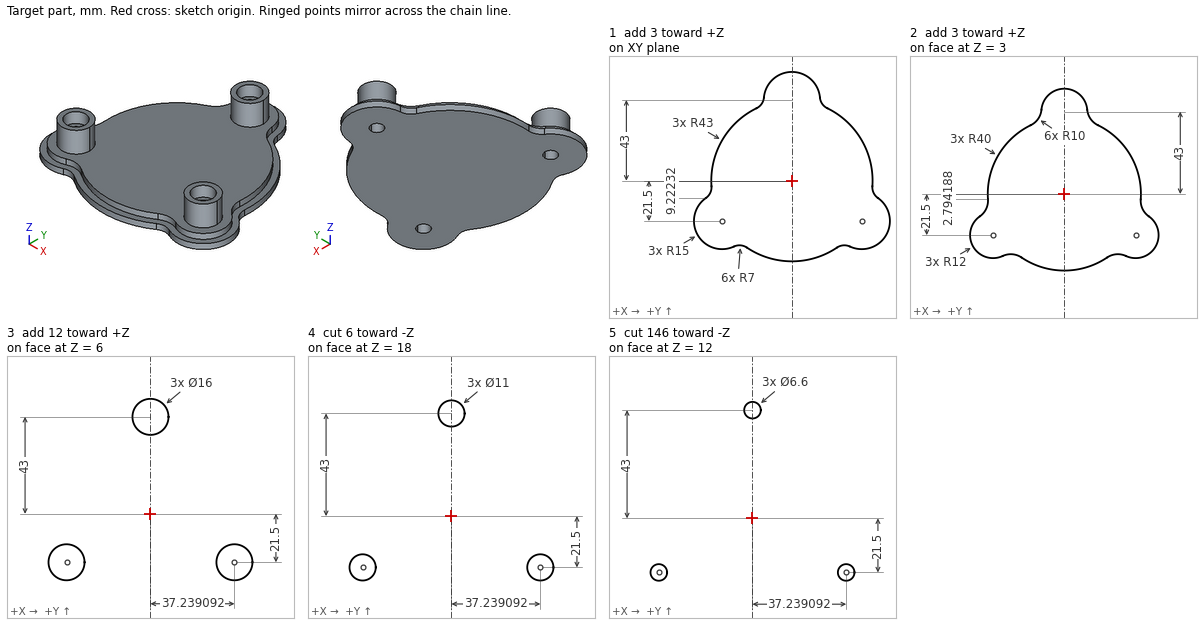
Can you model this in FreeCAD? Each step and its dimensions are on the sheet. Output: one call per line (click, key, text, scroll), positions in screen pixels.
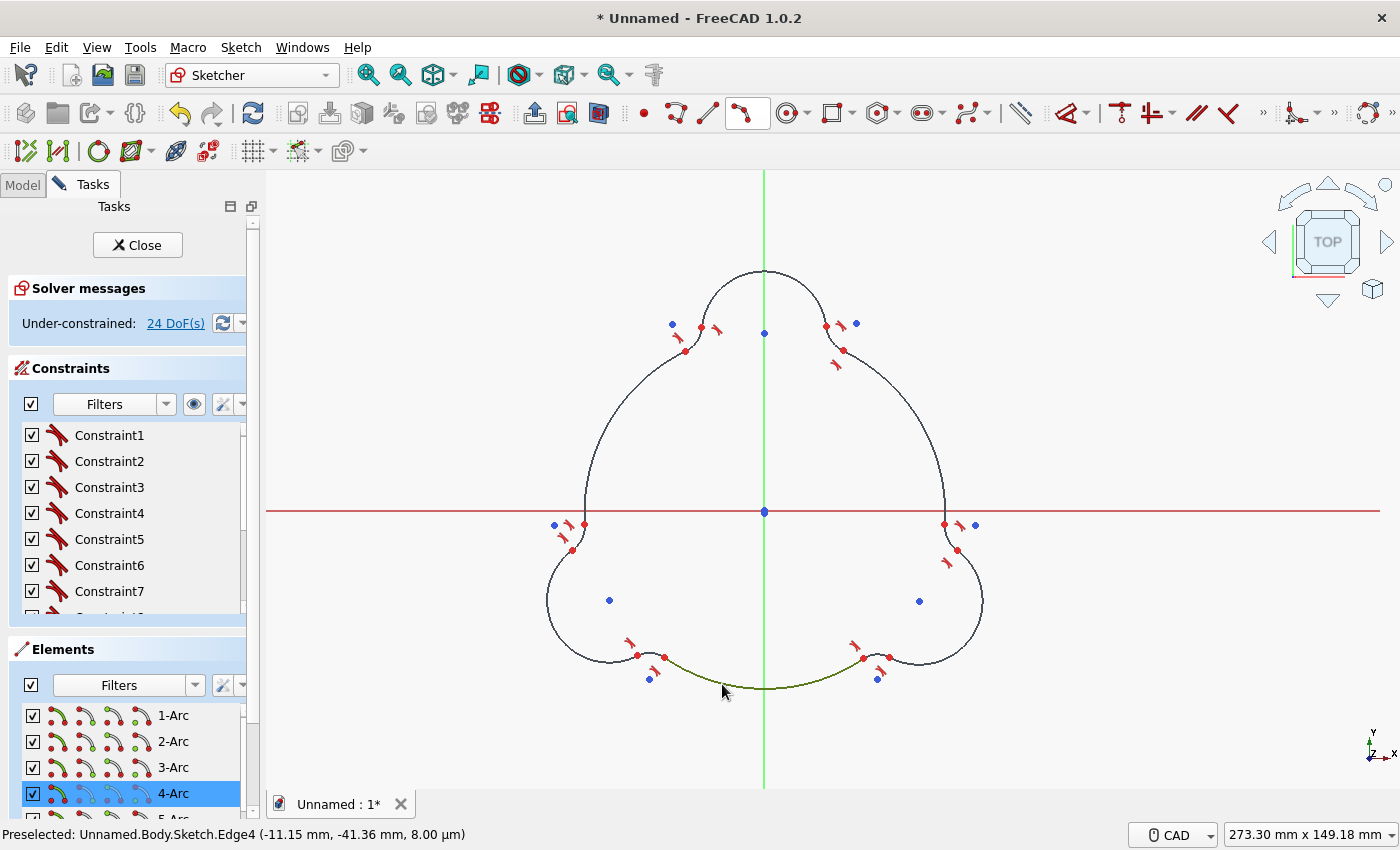
click(937, 461)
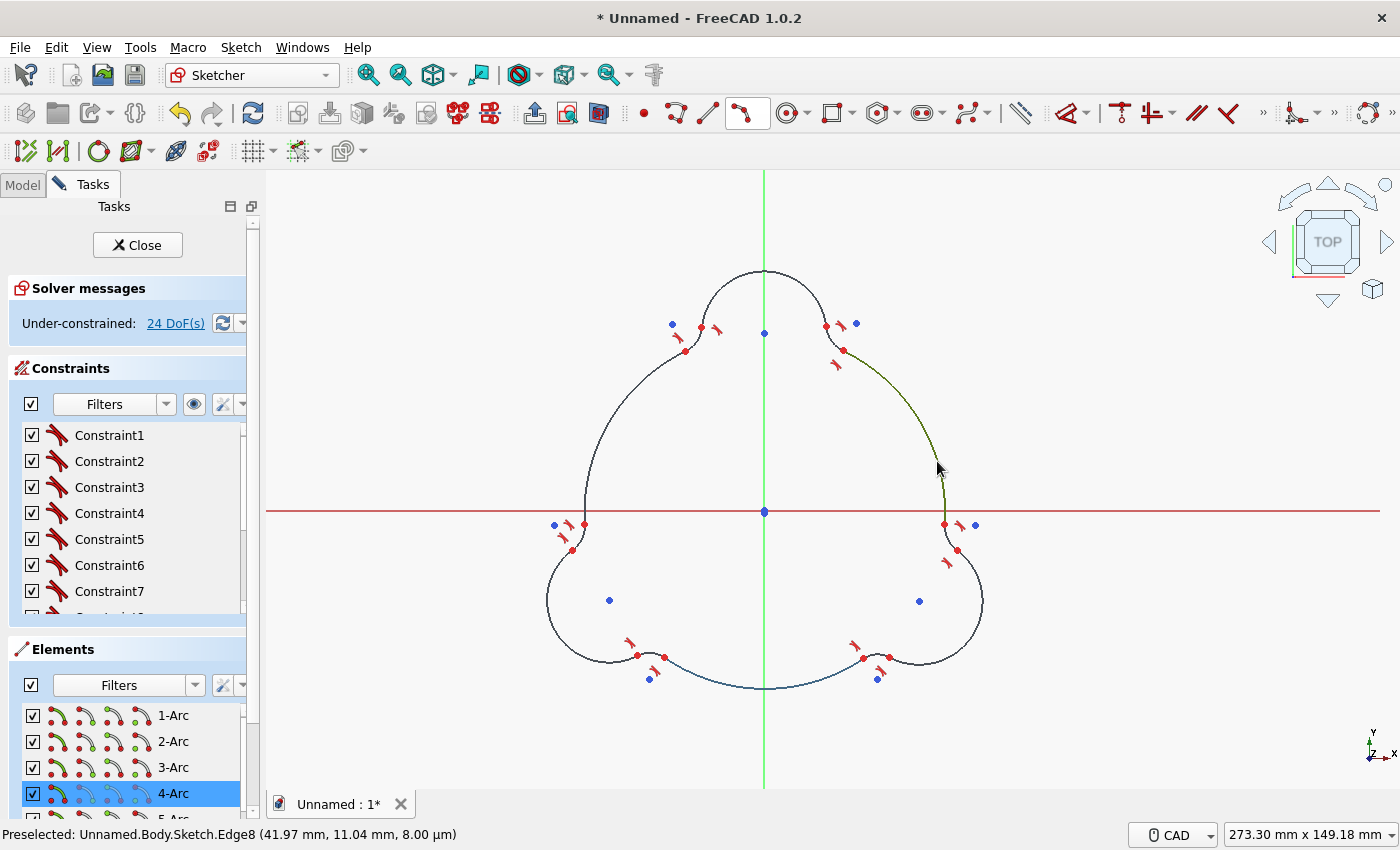
click(1120, 114)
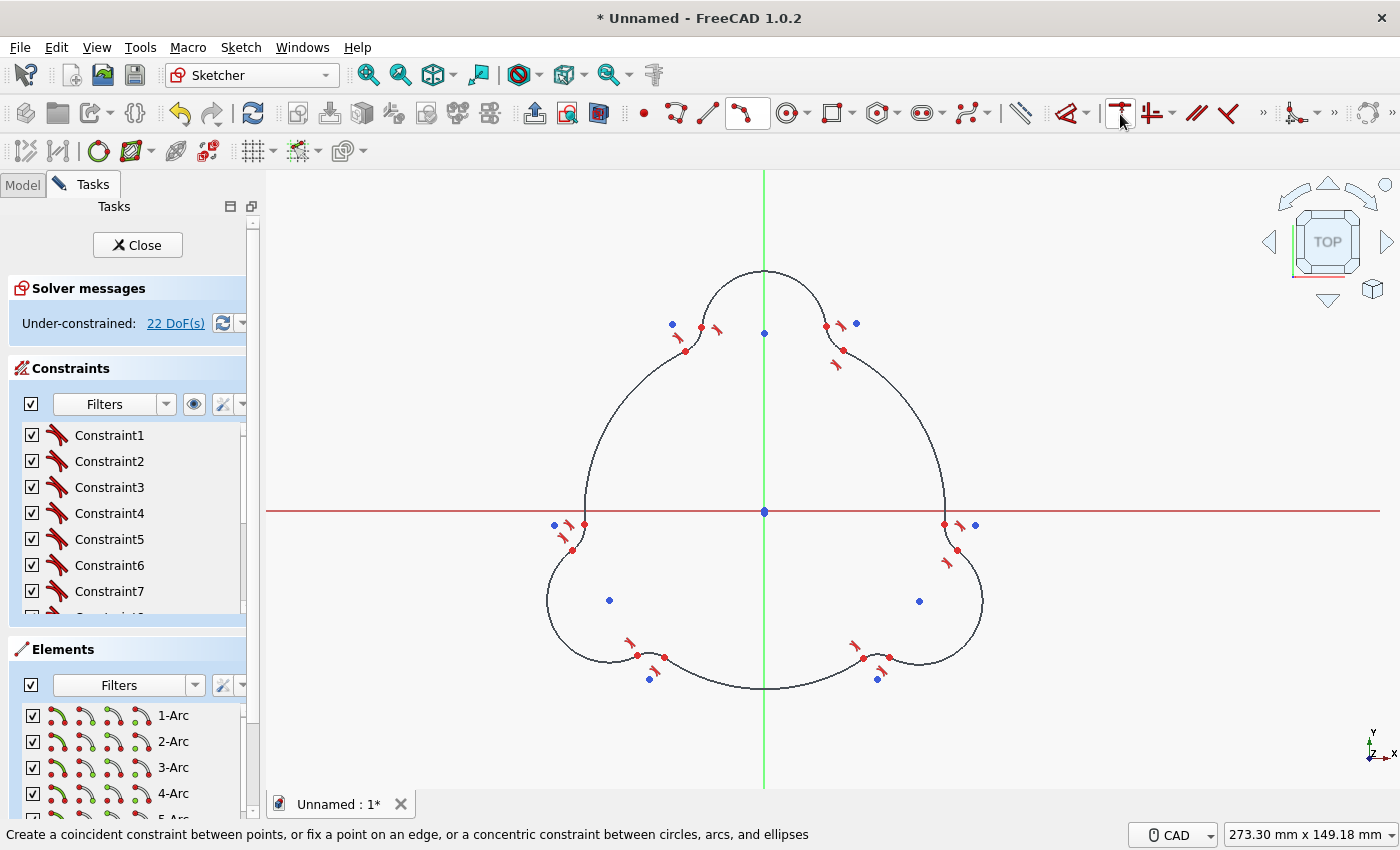
click(722, 684)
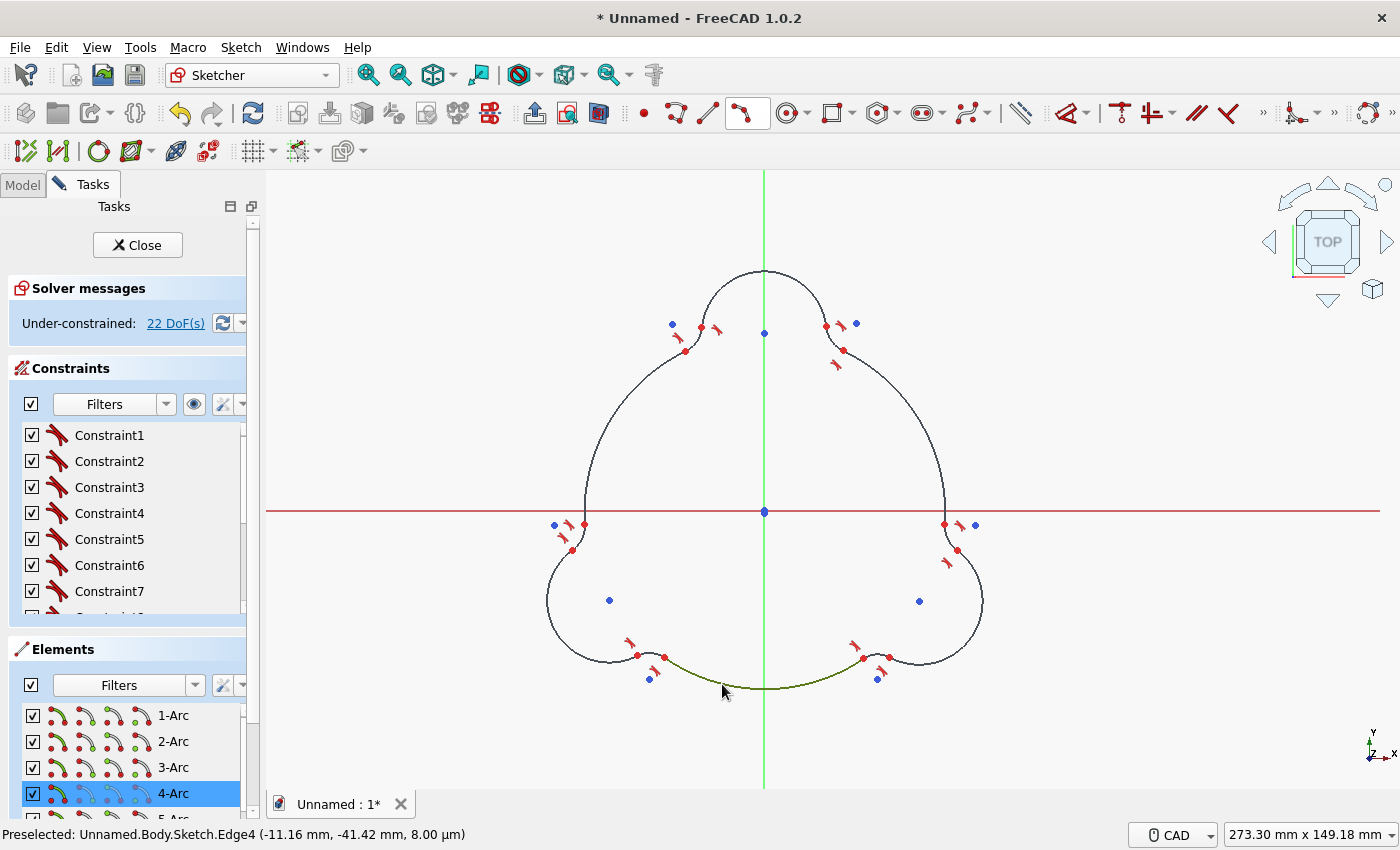
click(634, 389)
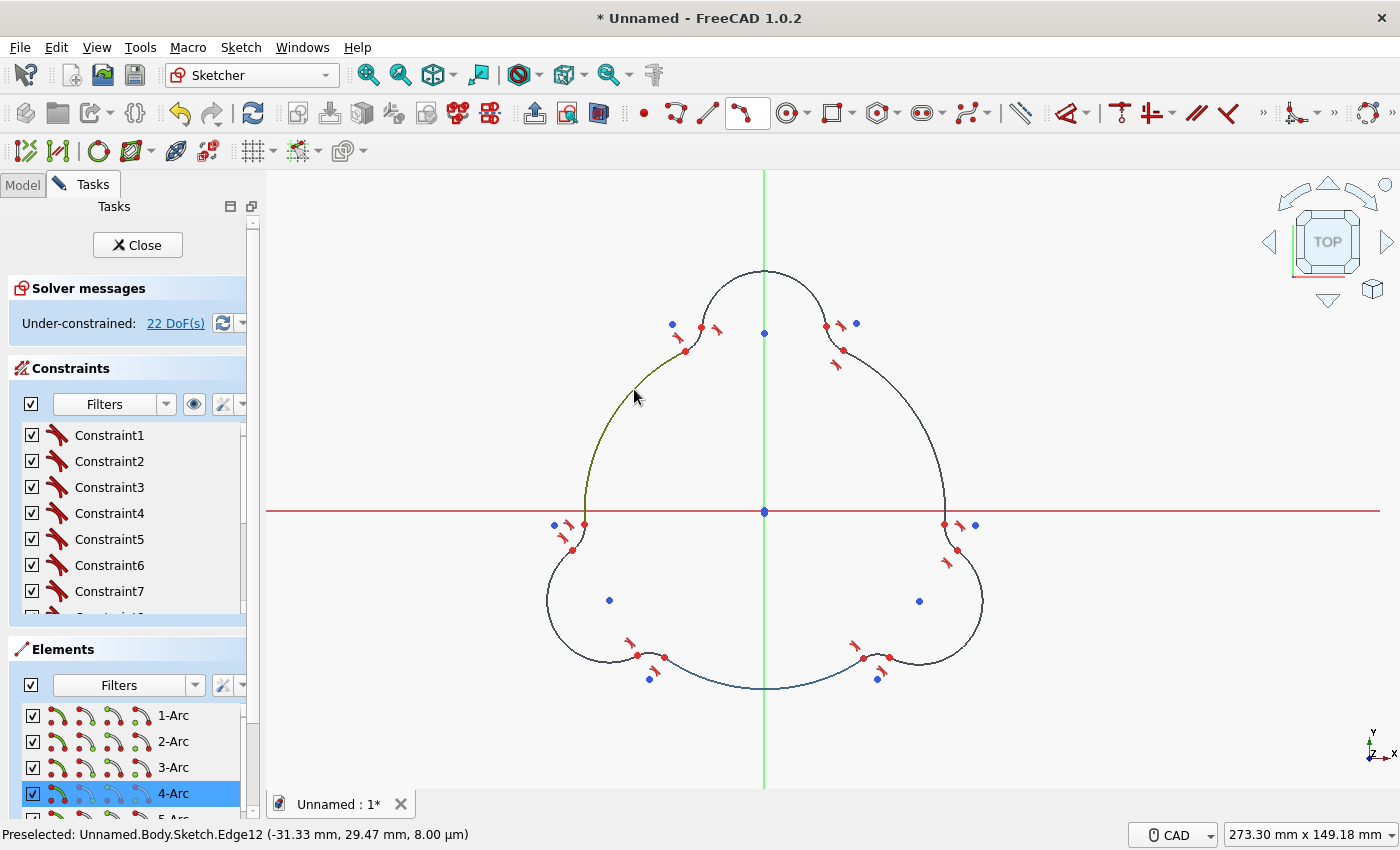
click(1120, 114)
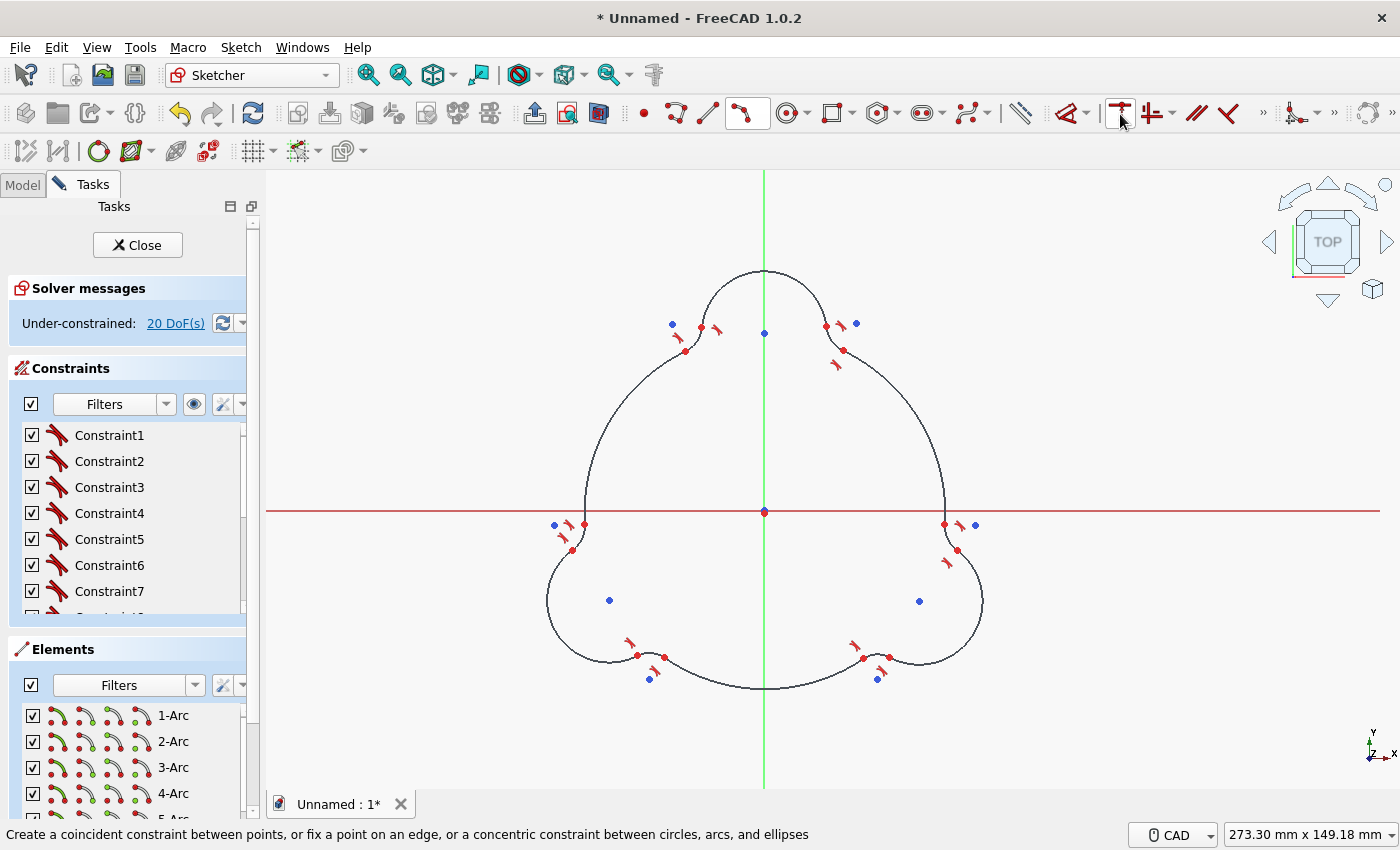
scroll(765, 512, up, 3)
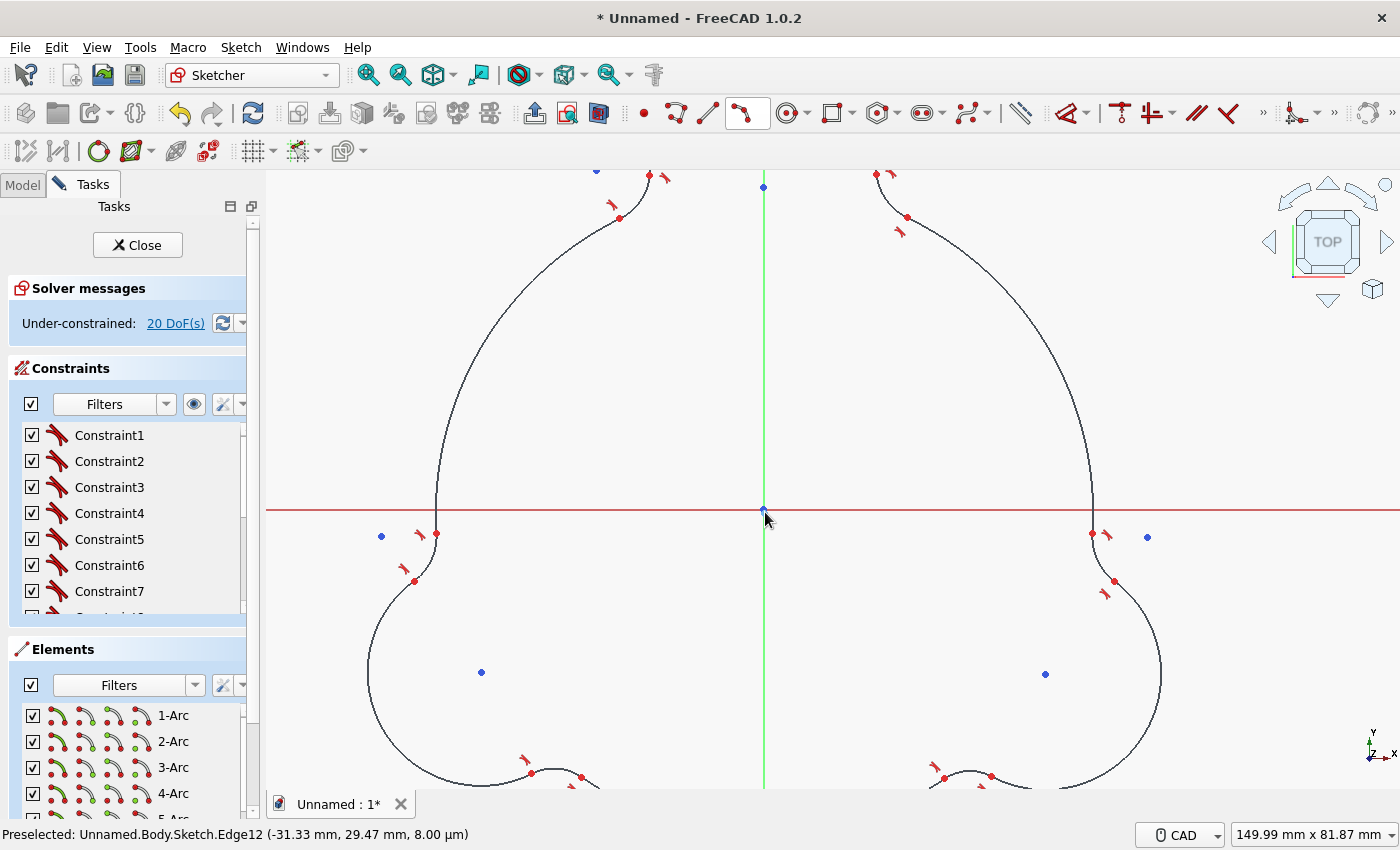
drag(754, 500, 774, 524)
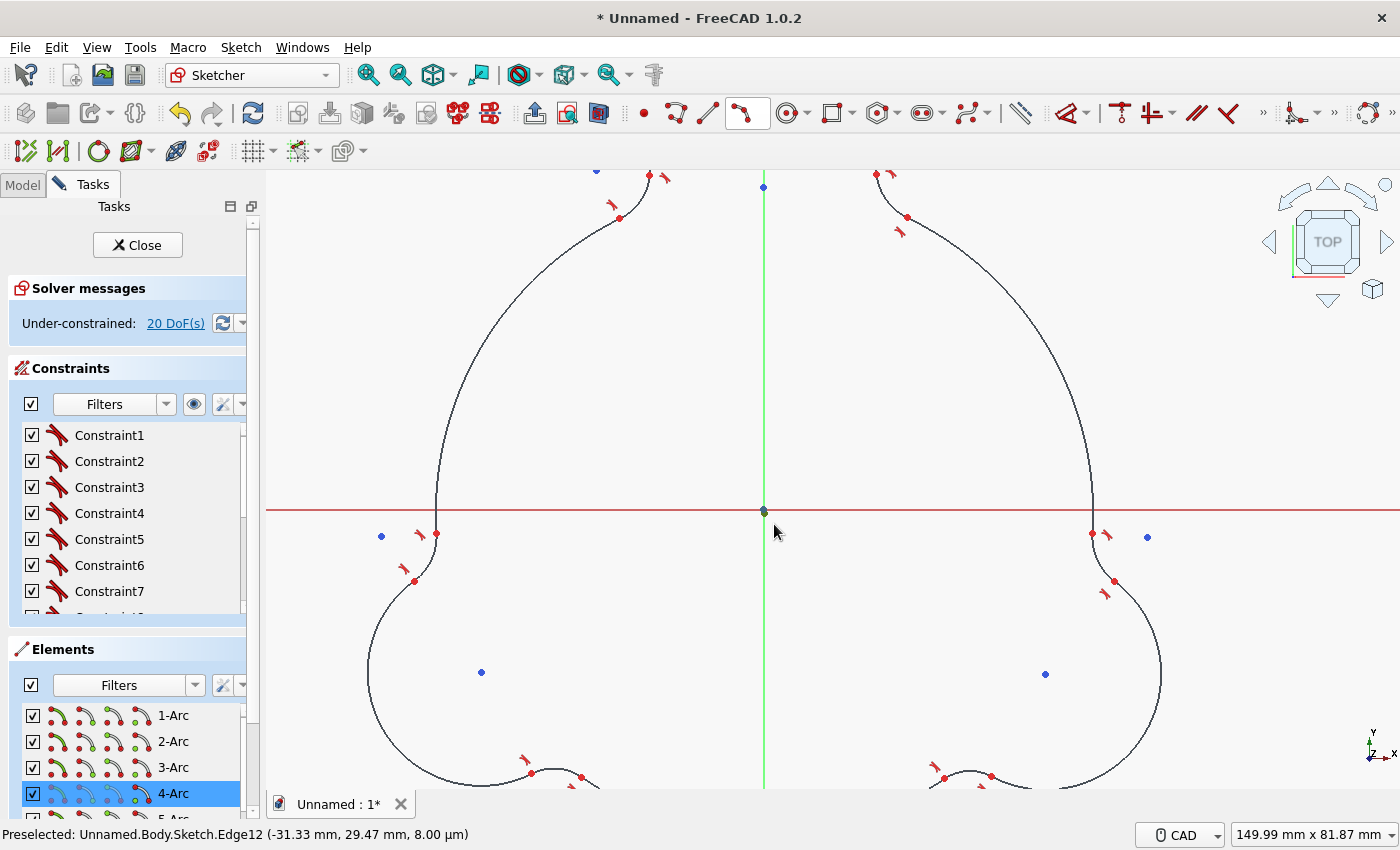
click(1120, 114)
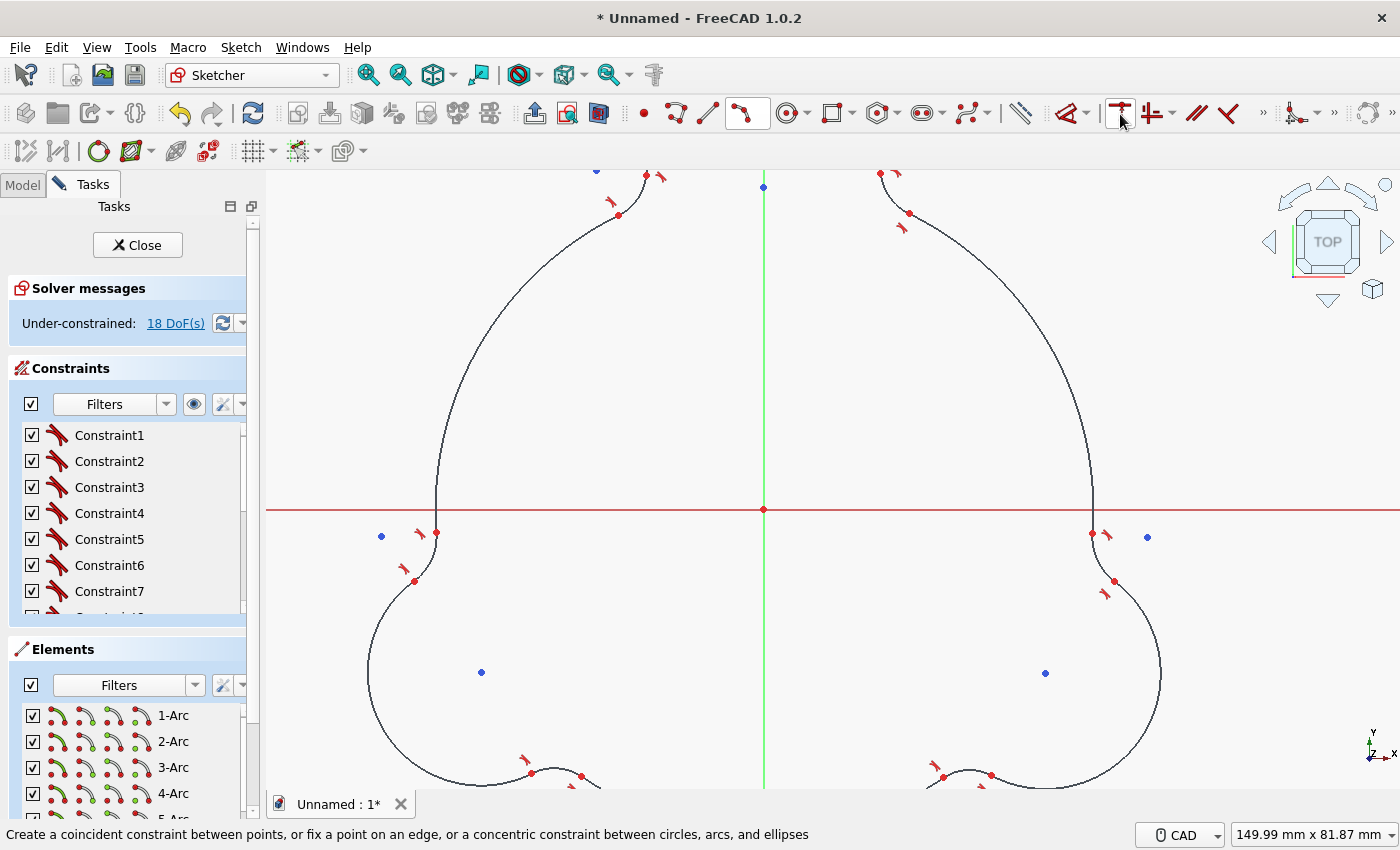
click(426, 569)